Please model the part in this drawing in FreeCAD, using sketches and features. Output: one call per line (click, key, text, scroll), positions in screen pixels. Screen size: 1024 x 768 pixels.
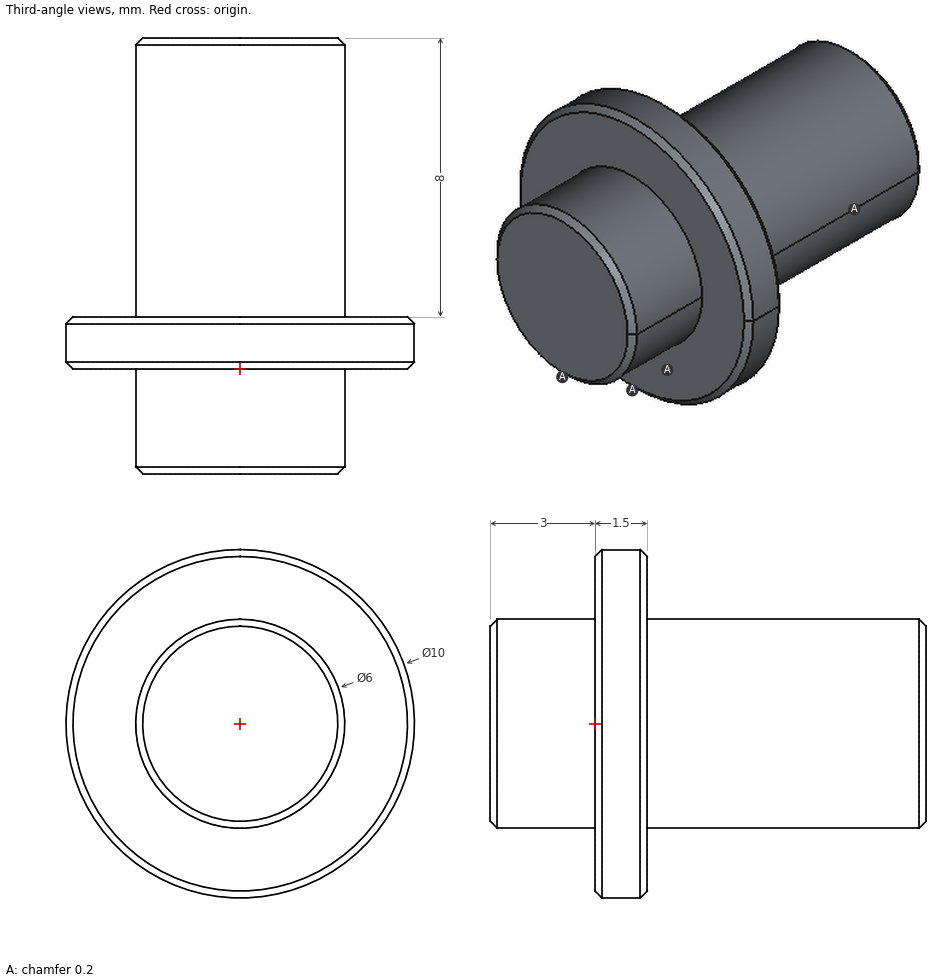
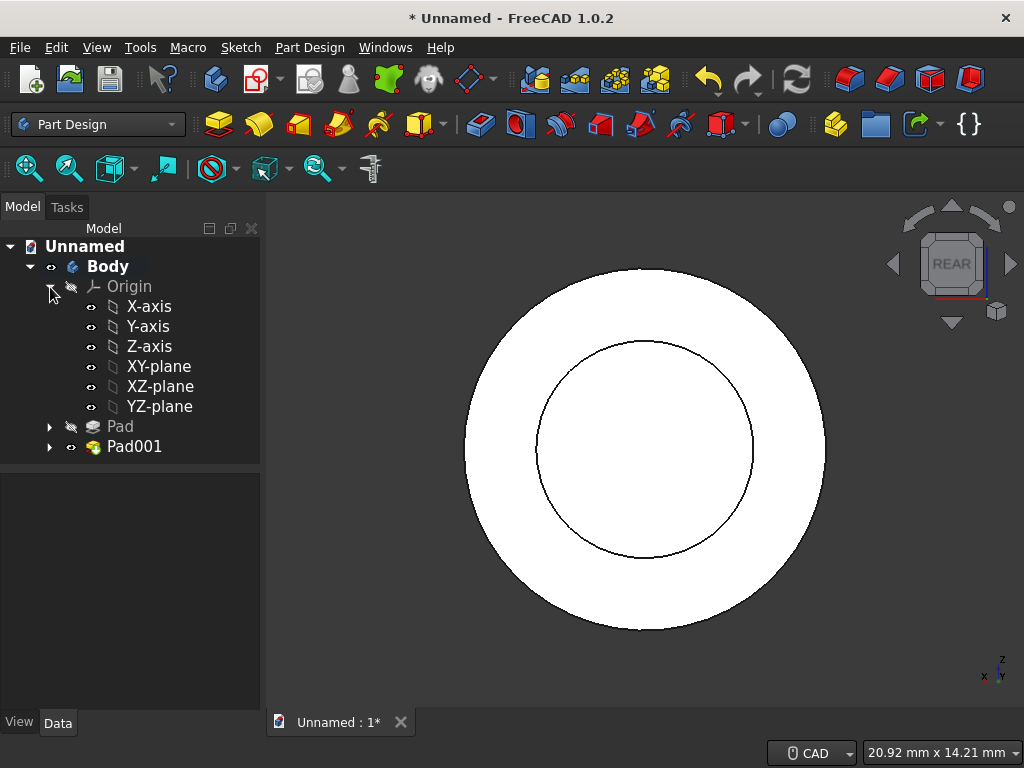
click(136, 387)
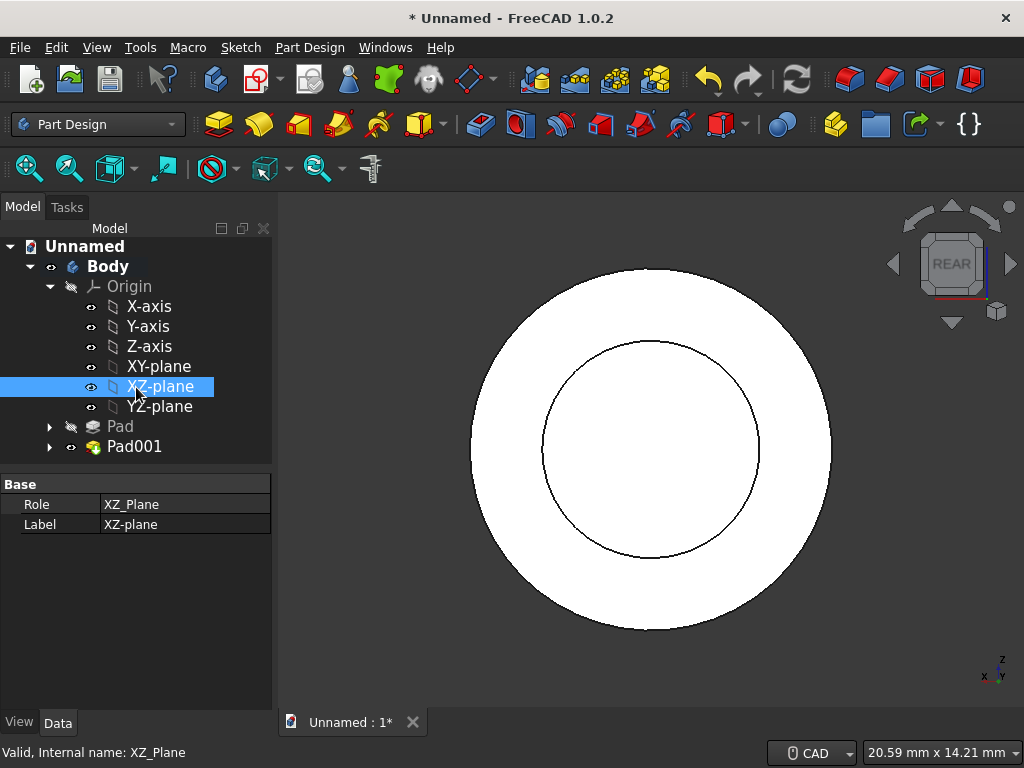
click(470, 80)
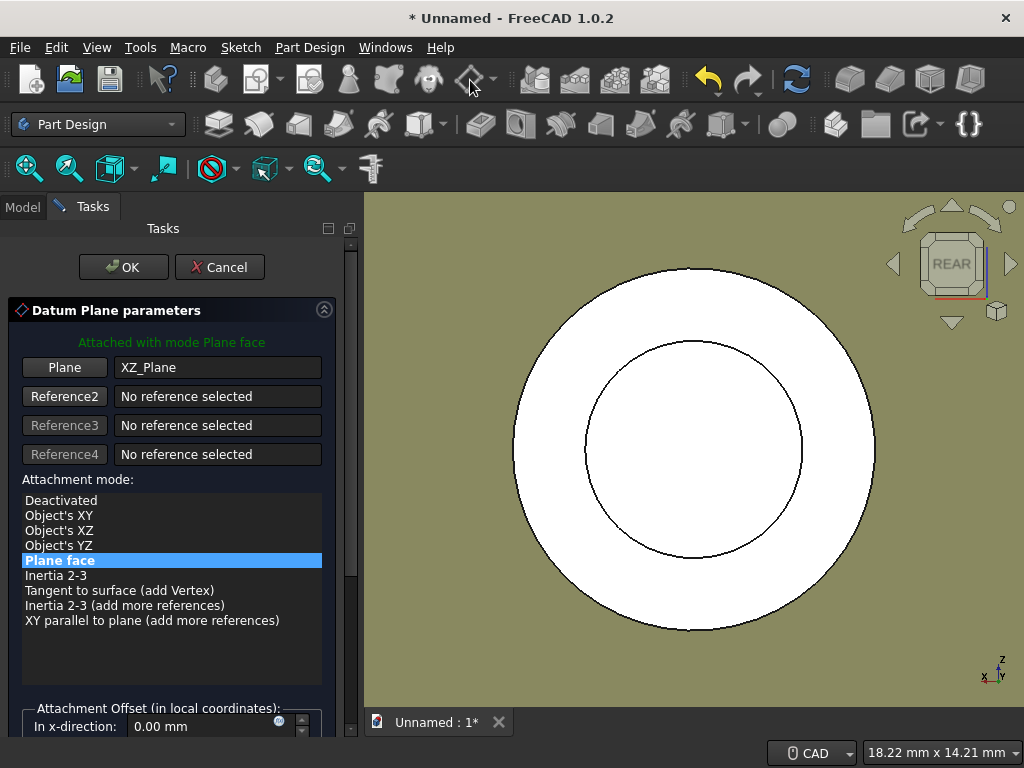
scroll(351, 487, down, 3)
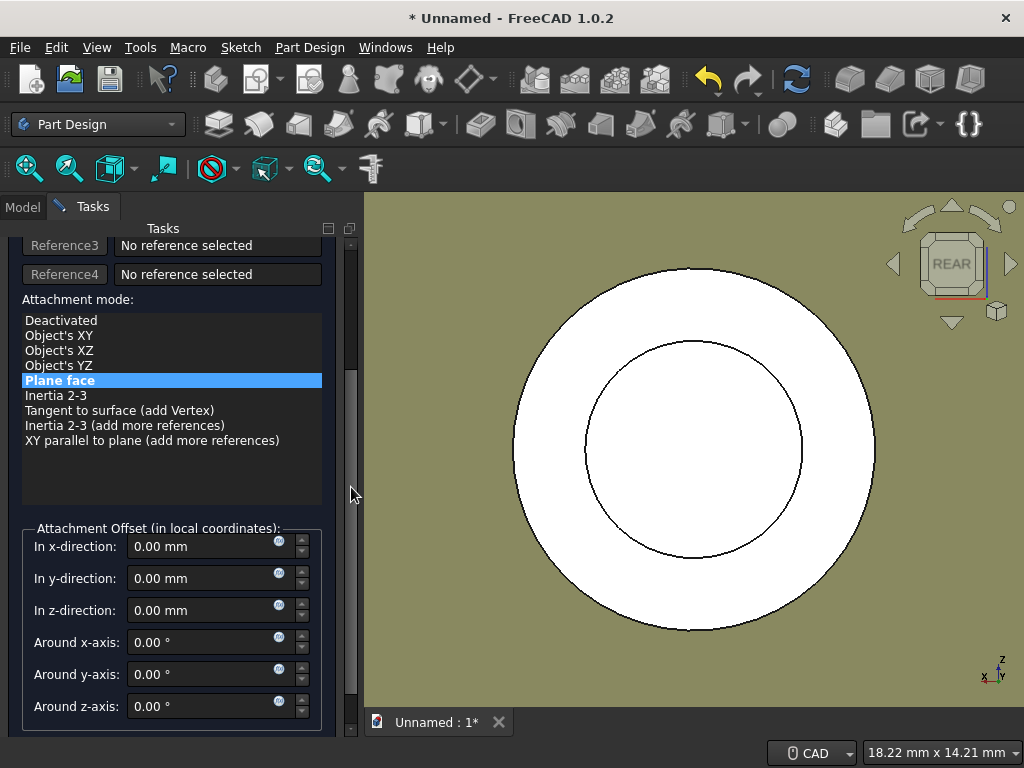
triple_click(210, 610)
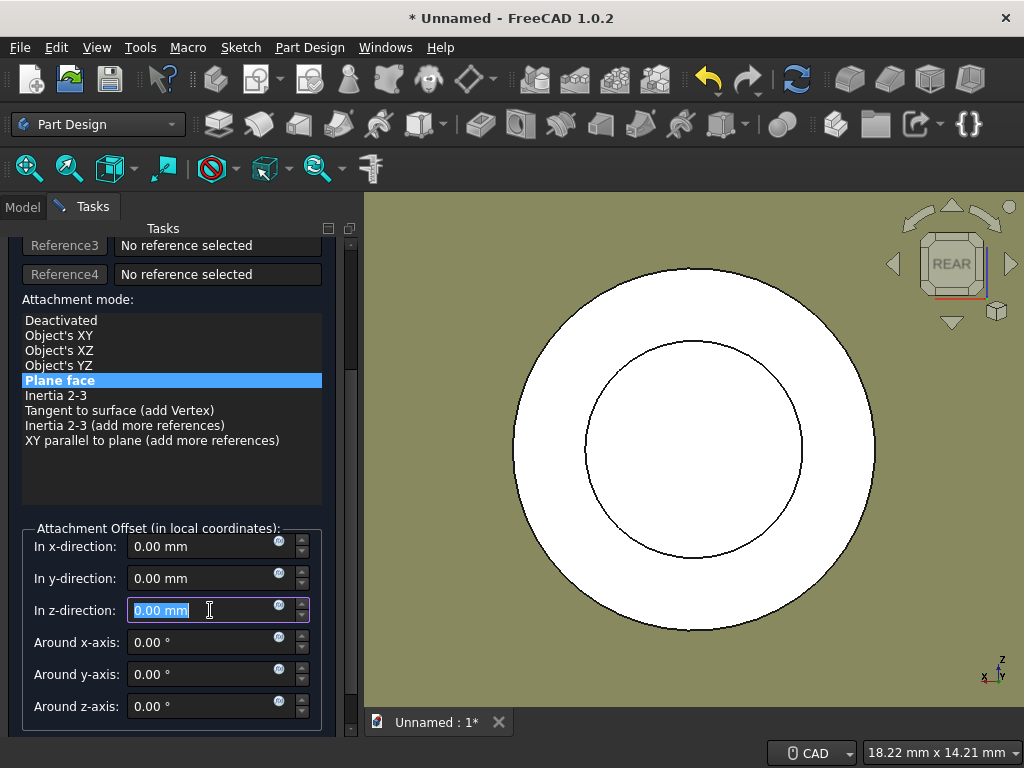
text(3)
key(Tab)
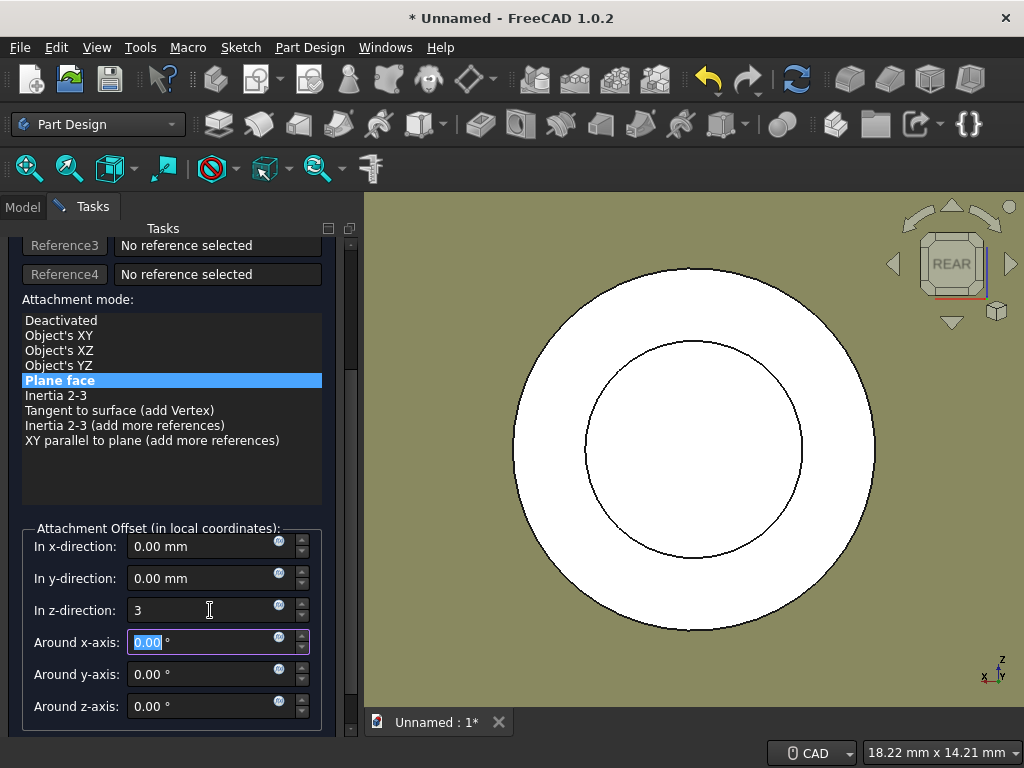
scroll(351, 487, up, 4)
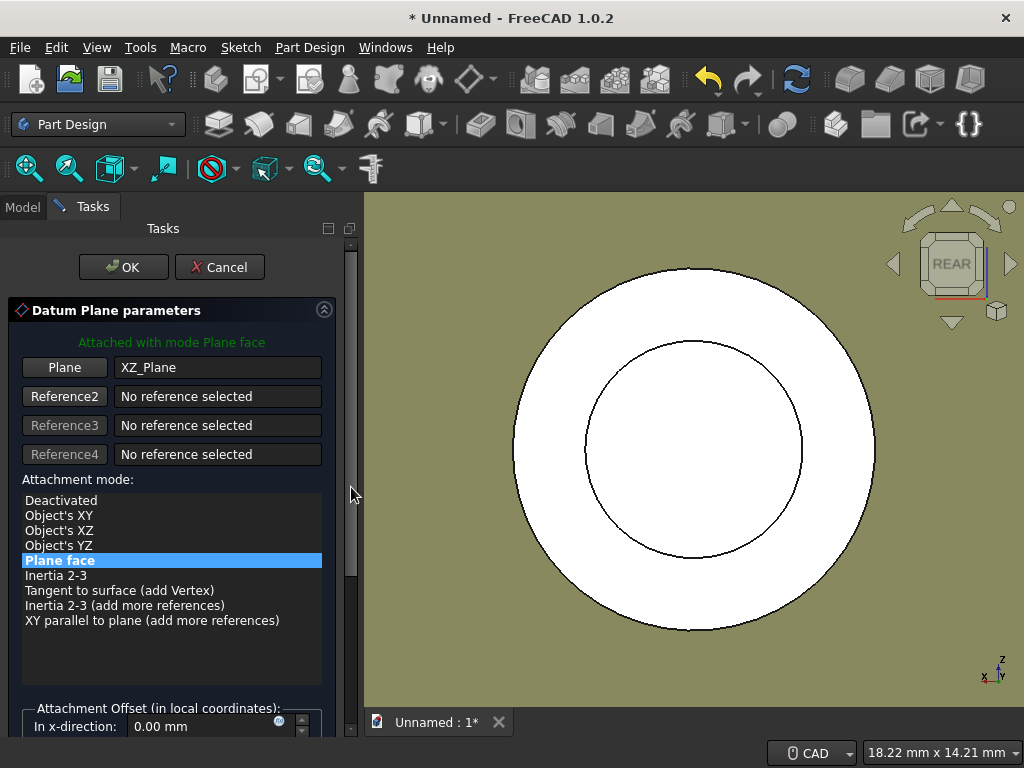
click(124, 267)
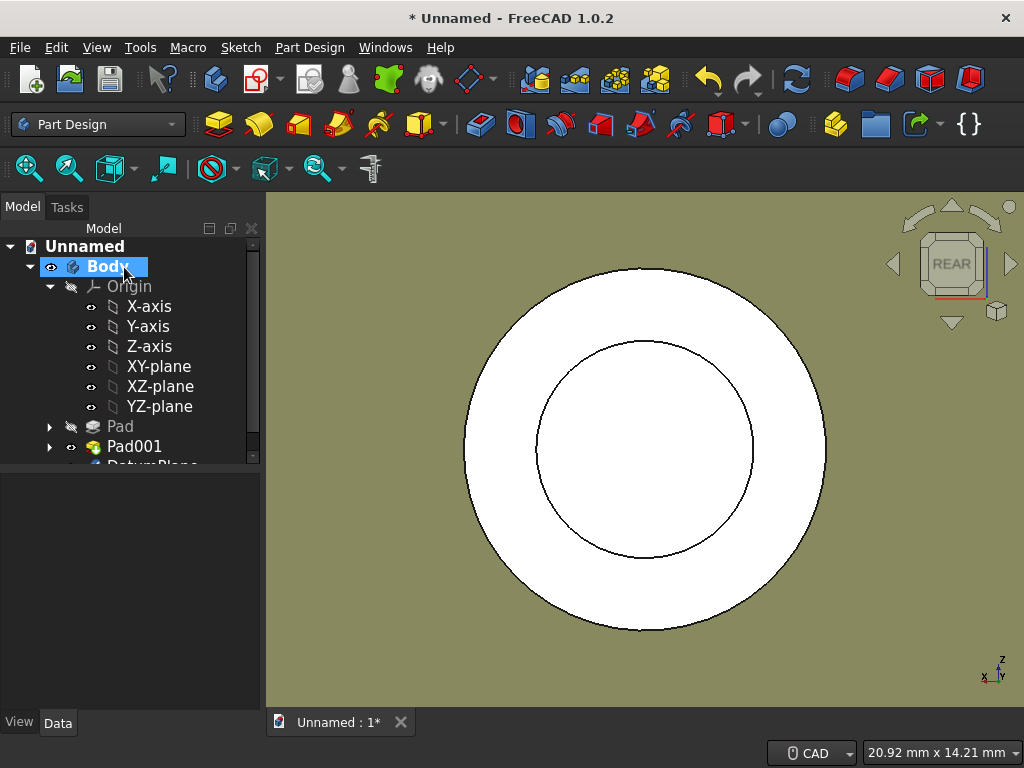
scroll(100, 342, down, 3)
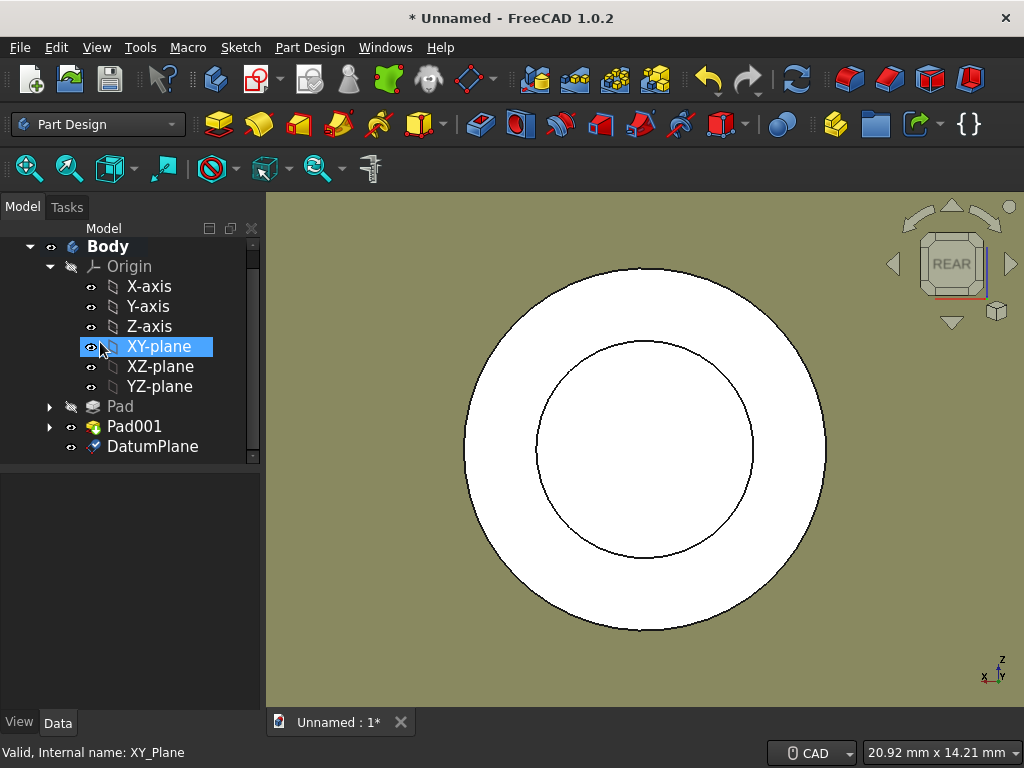
click(116, 447)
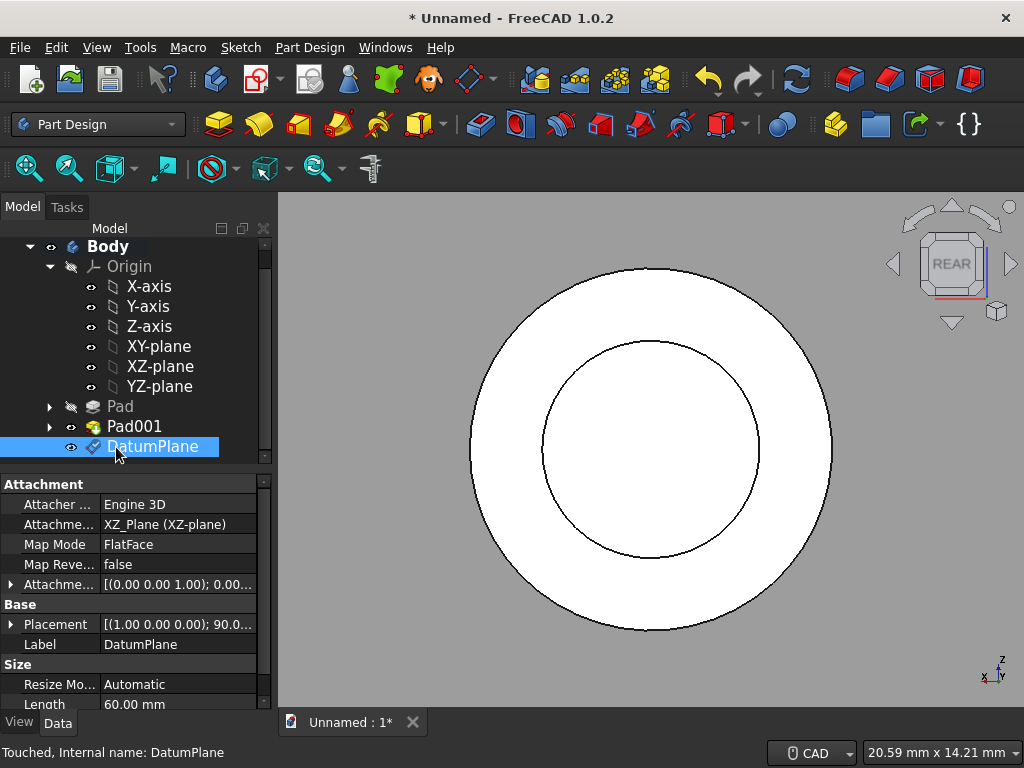
click(256, 80)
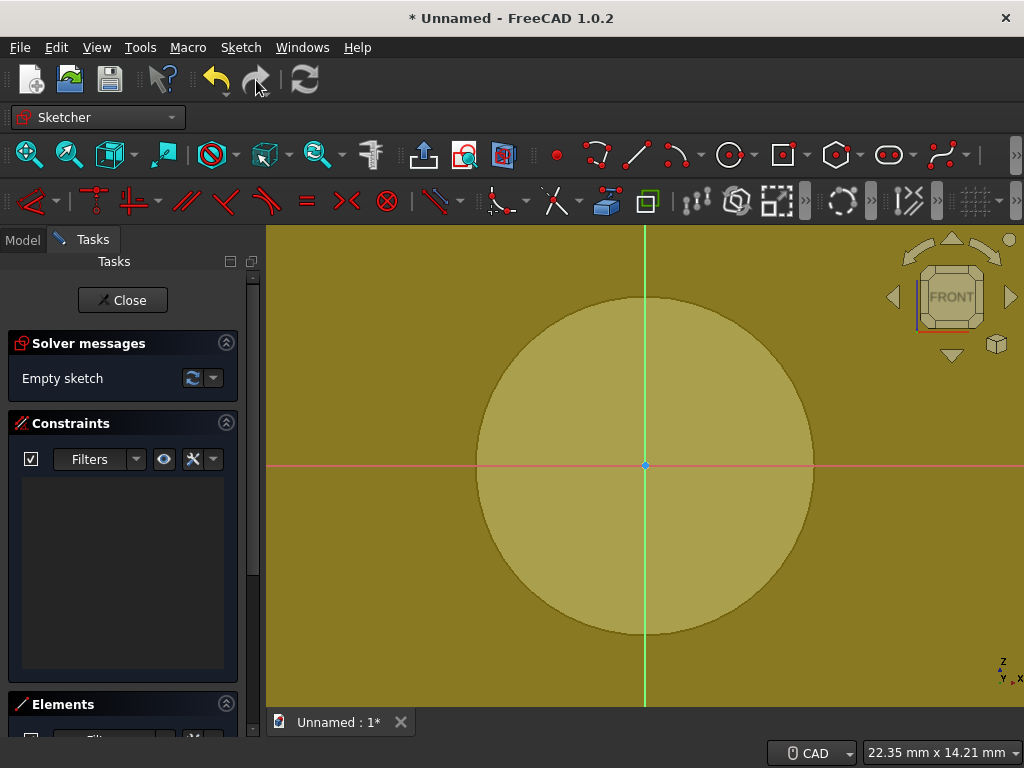
scroll(784, 466, up, 2)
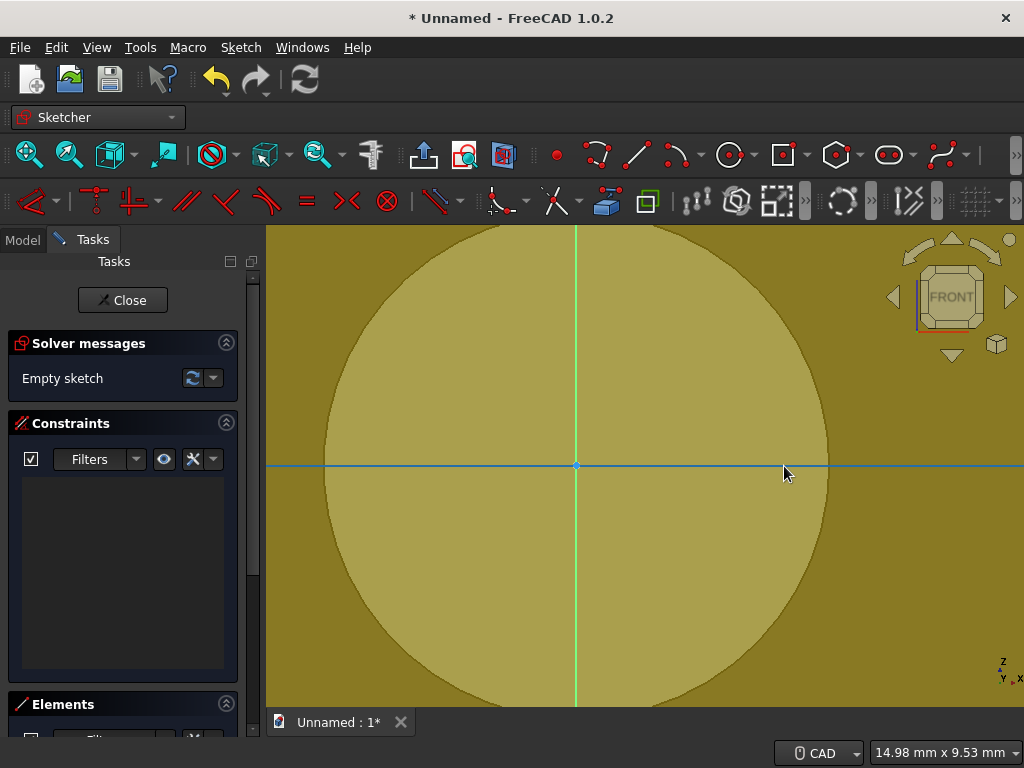
key(g)
key(c)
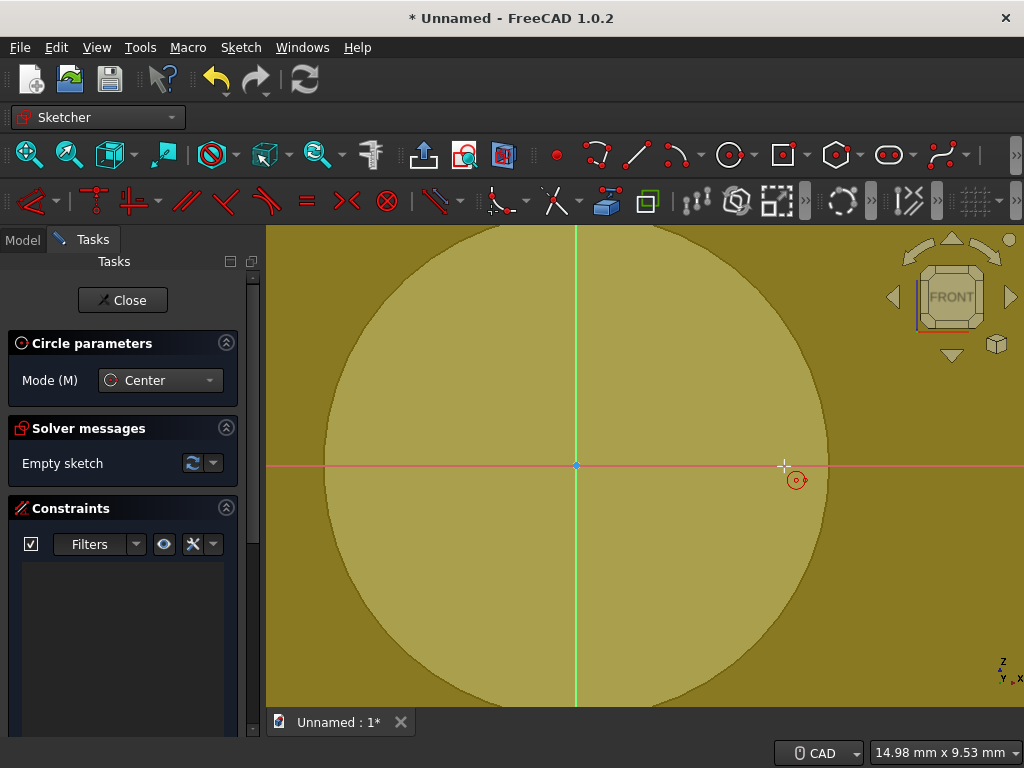
click(576, 466)
move(684, 358)